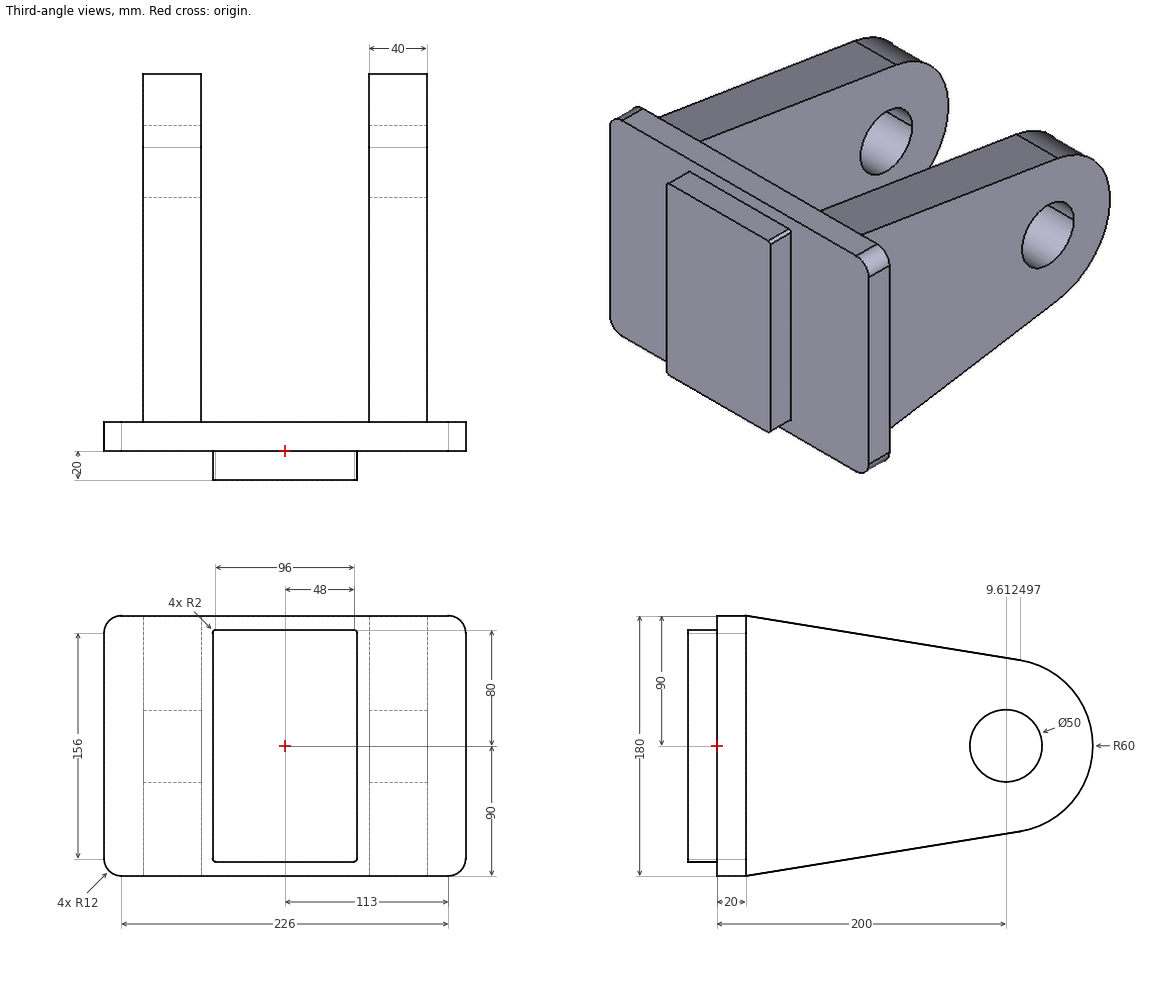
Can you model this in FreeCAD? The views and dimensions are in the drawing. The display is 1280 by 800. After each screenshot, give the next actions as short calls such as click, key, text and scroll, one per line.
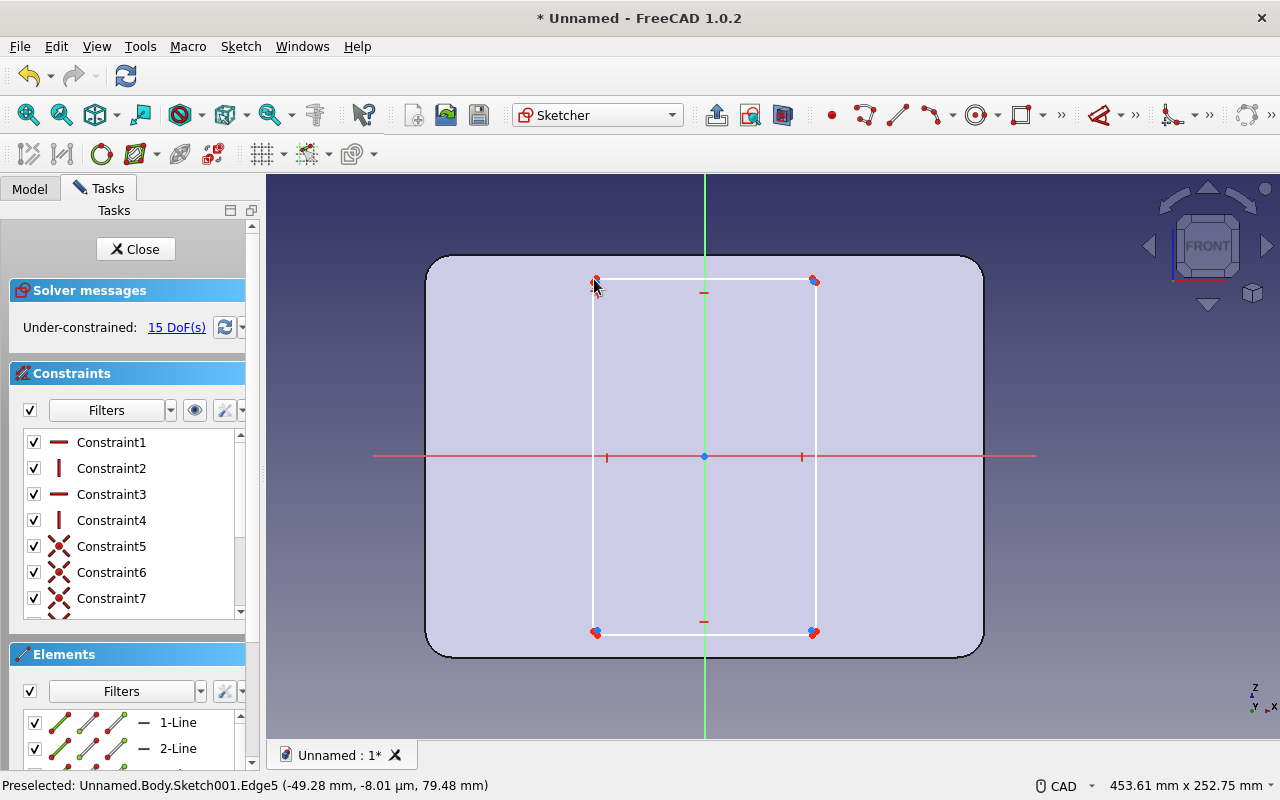
click(662, 279)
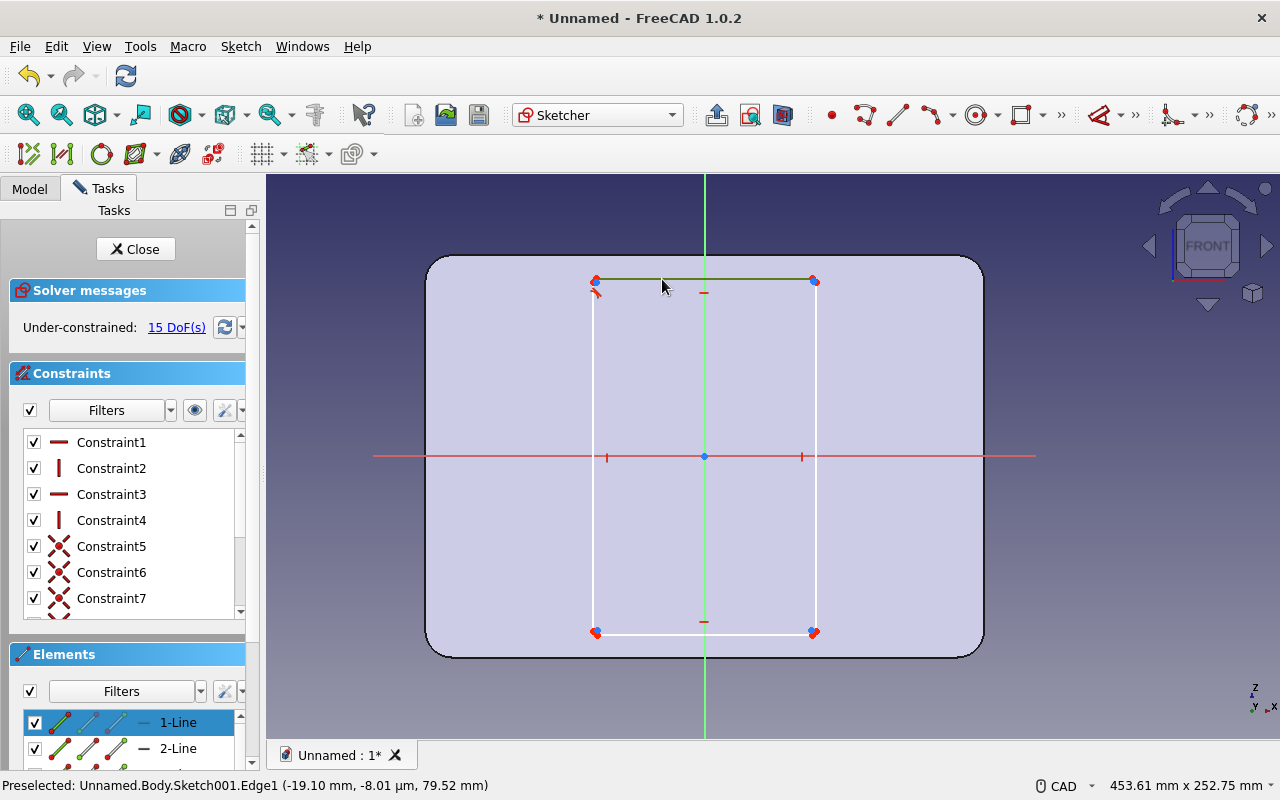
scroll(816, 279, up, 8)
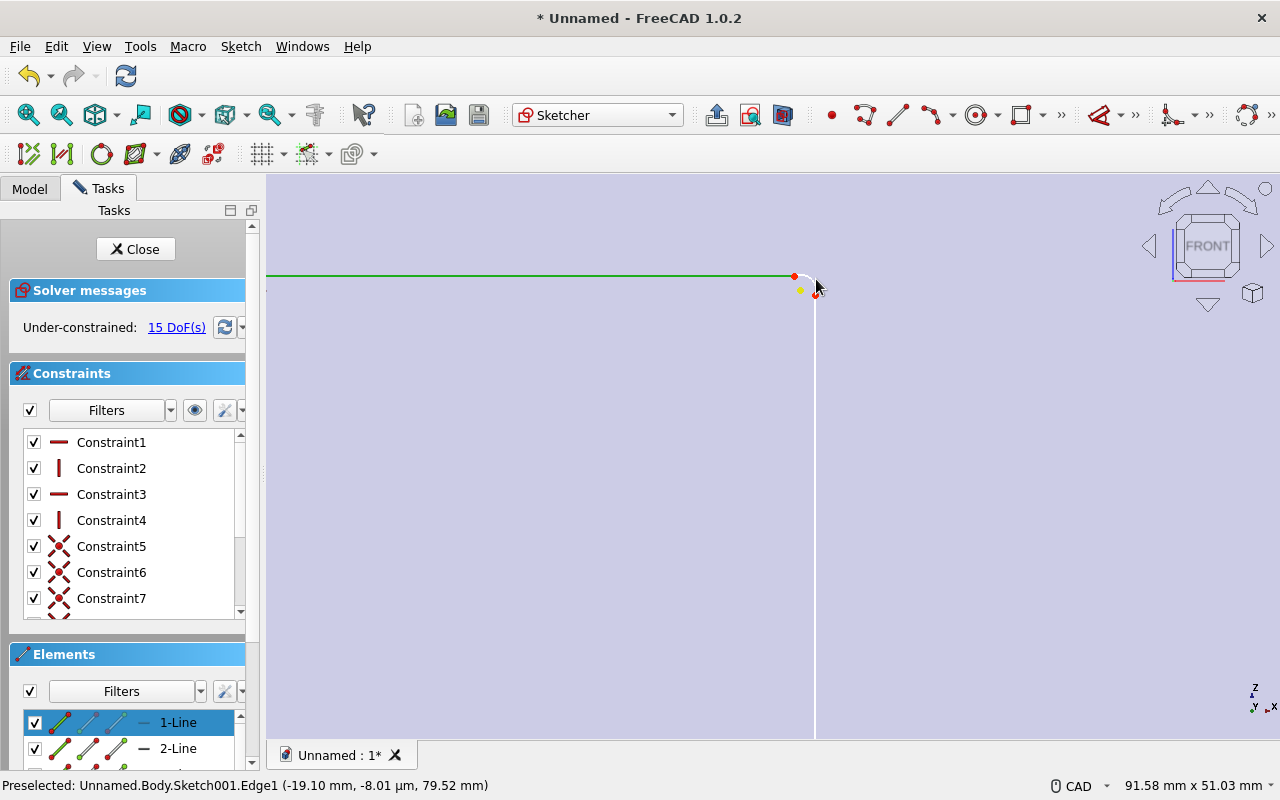
click(811, 279)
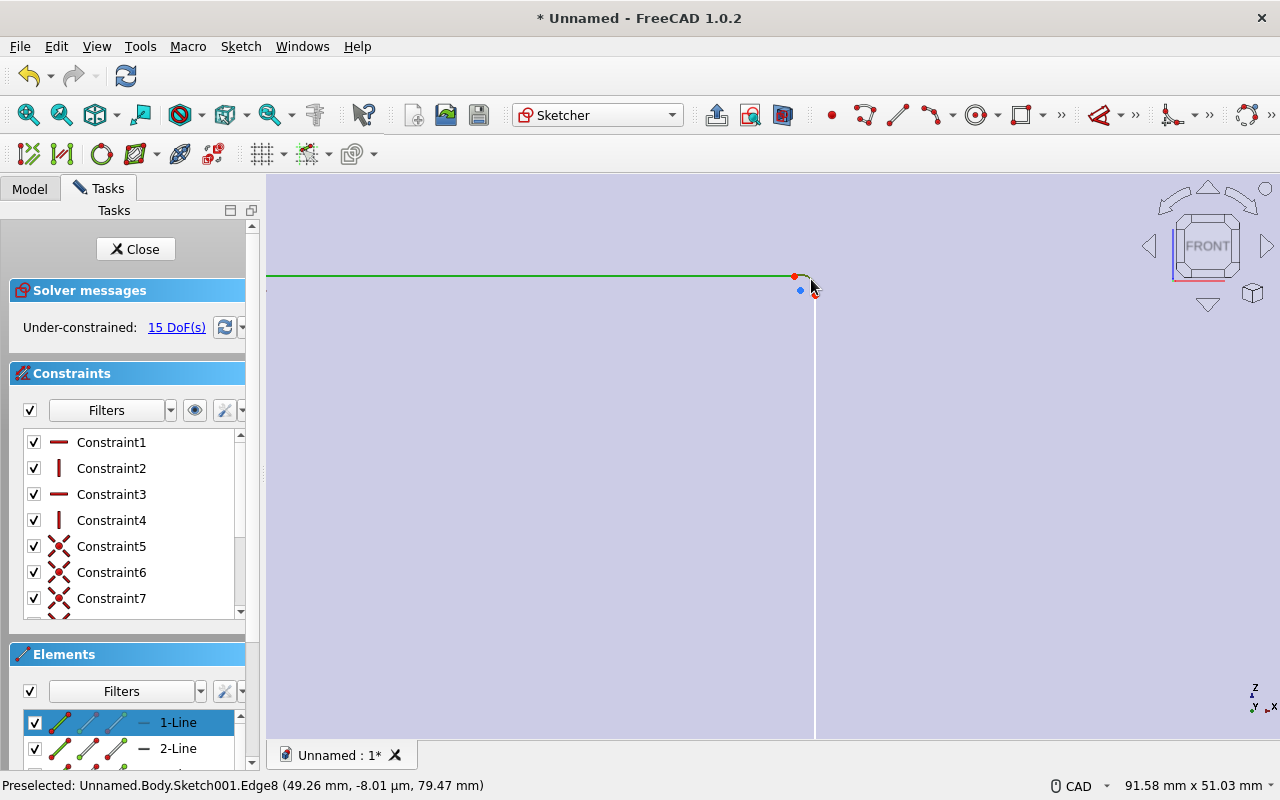
key(t)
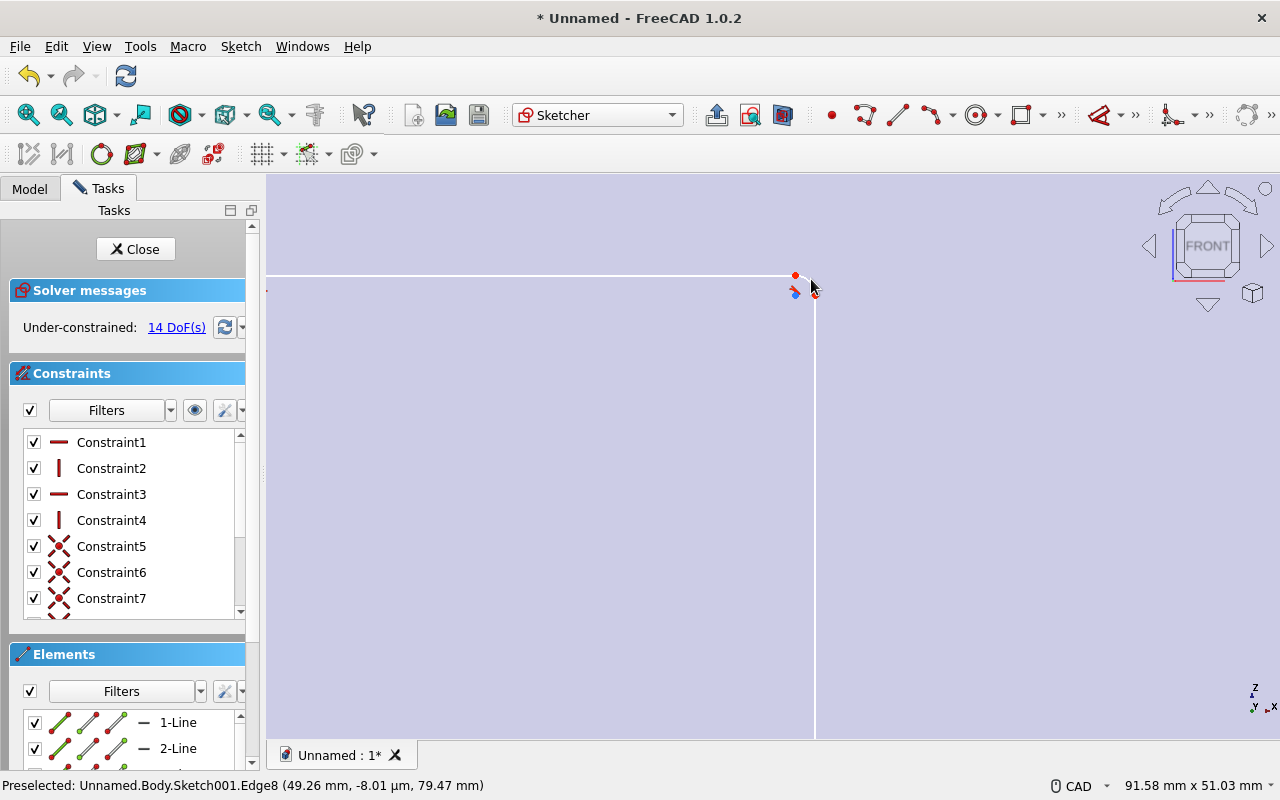
scroll(816, 279, down, 8)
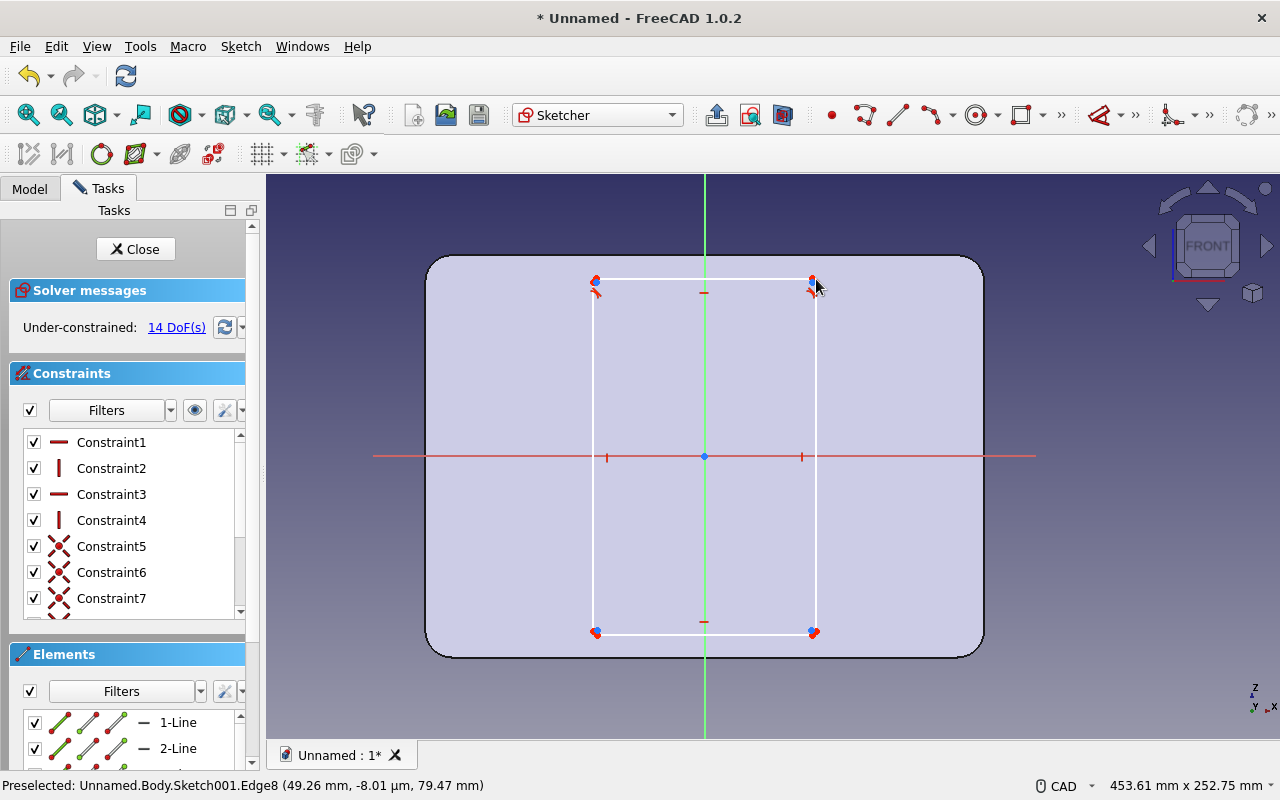
click(593, 387)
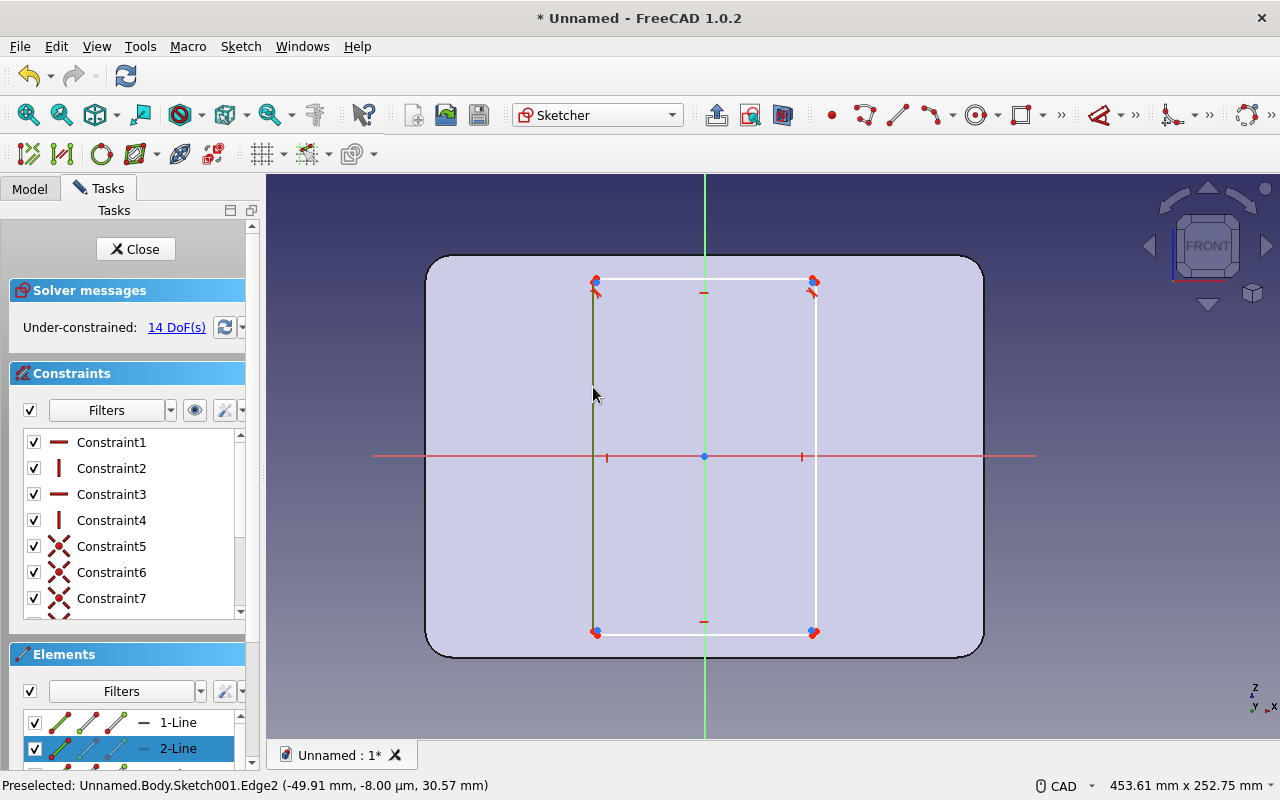
scroll(594, 280, up, 8)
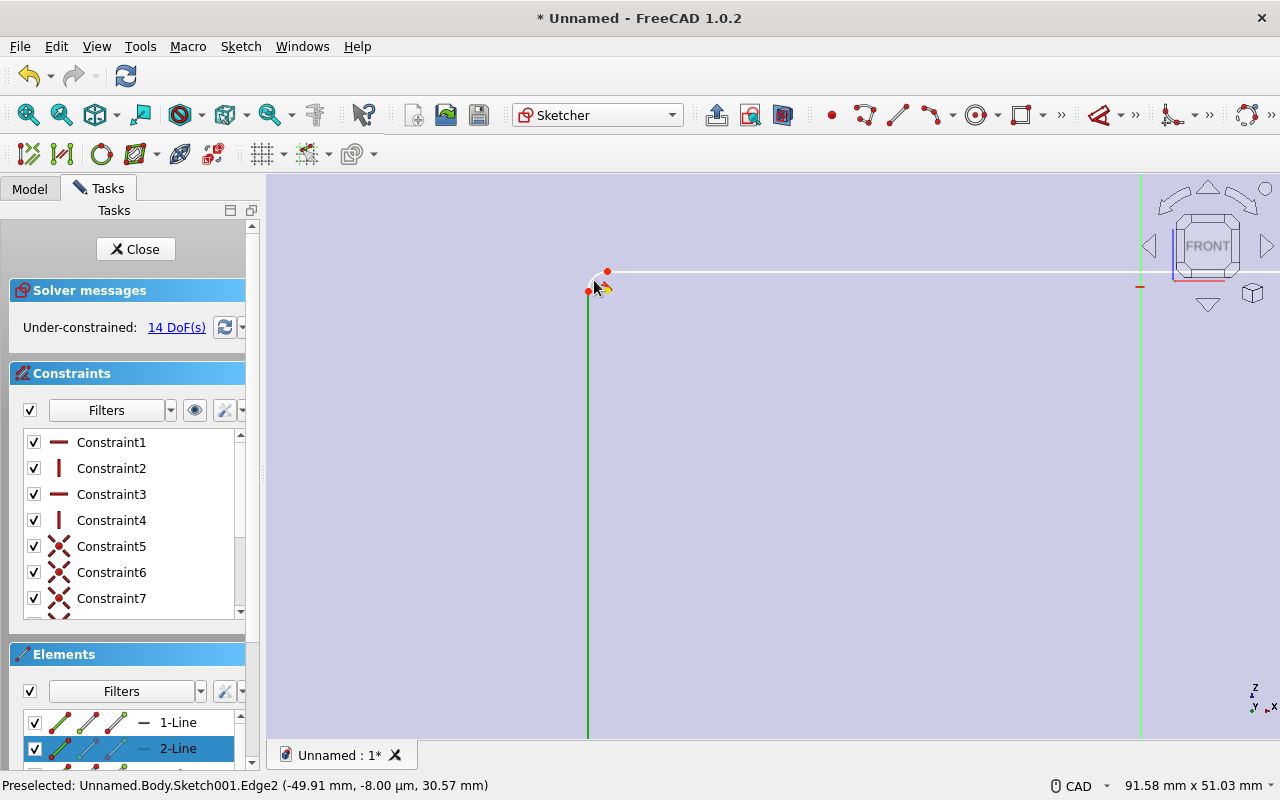
click(594, 278)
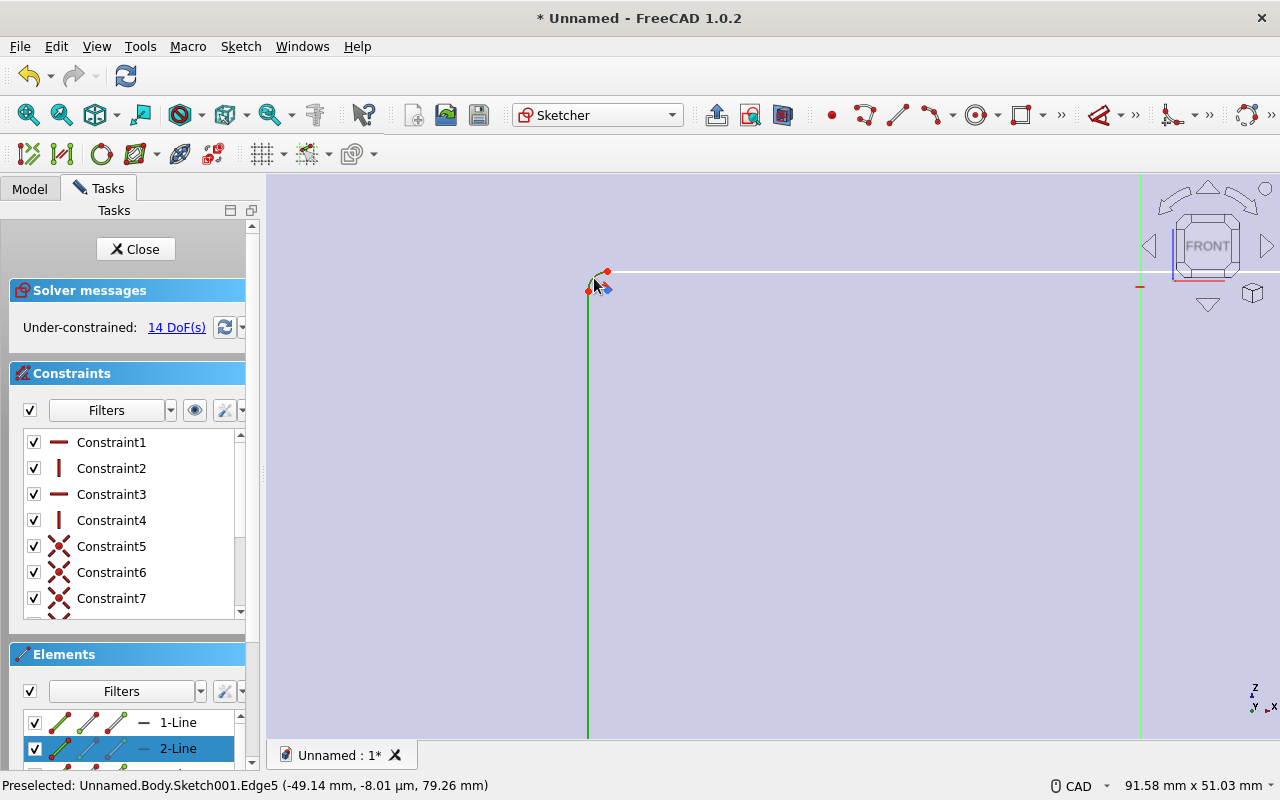
key(t)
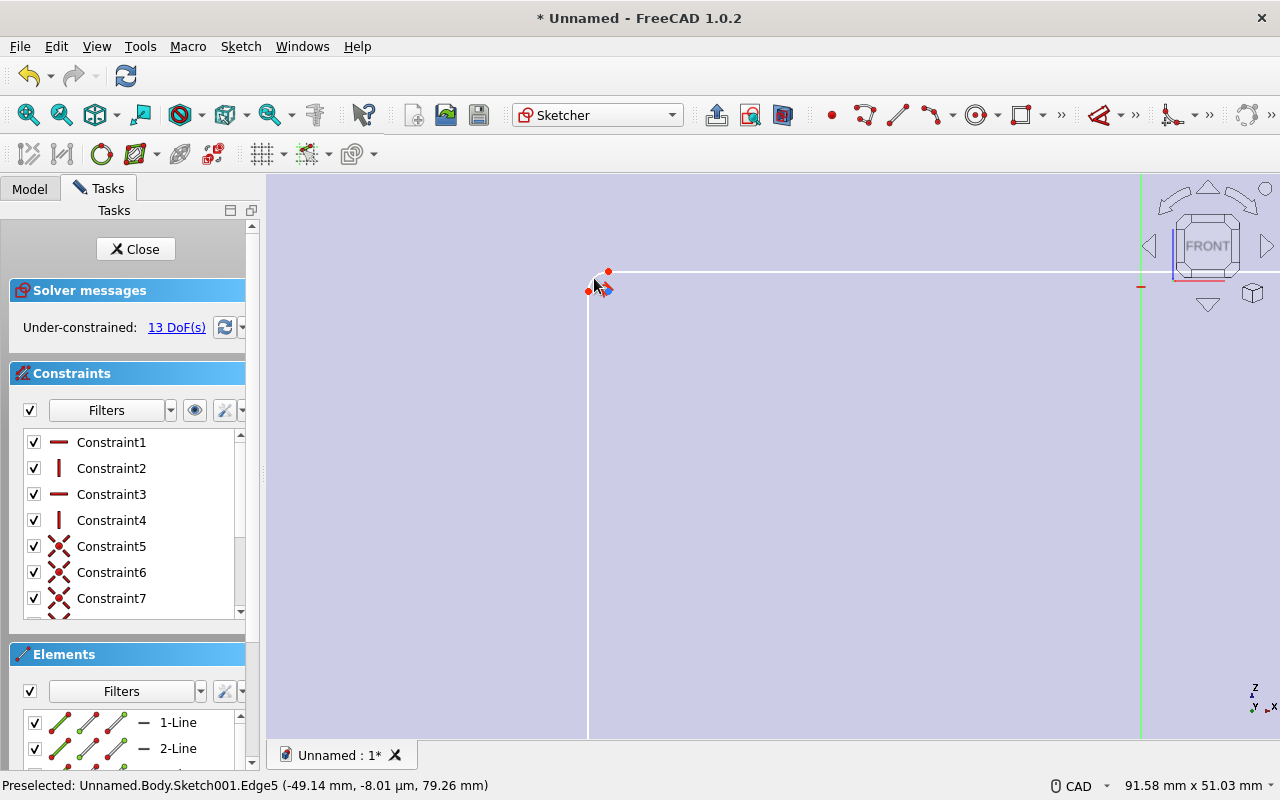
scroll(594, 280, down, 8)